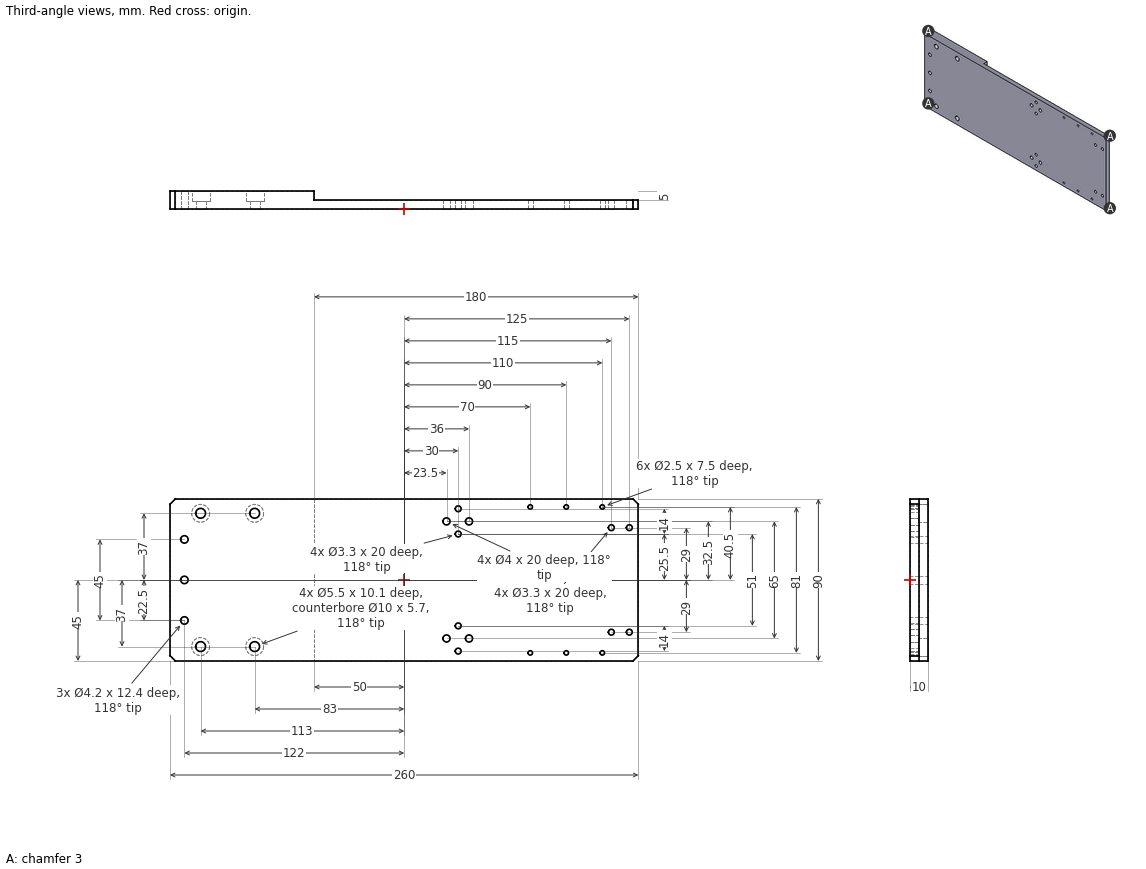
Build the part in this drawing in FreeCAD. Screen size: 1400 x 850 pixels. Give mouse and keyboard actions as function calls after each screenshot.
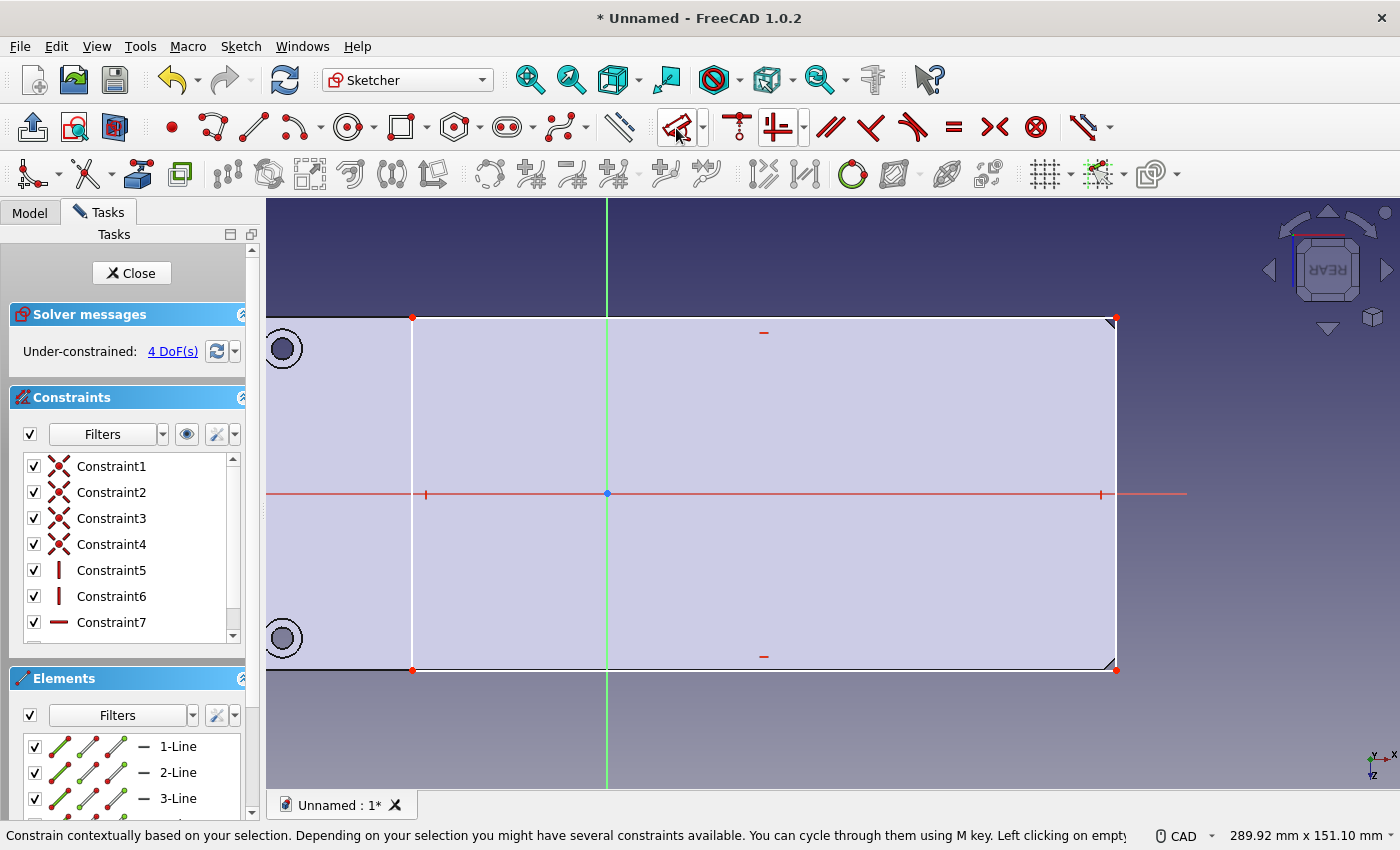
click(412, 424)
click(378, 413)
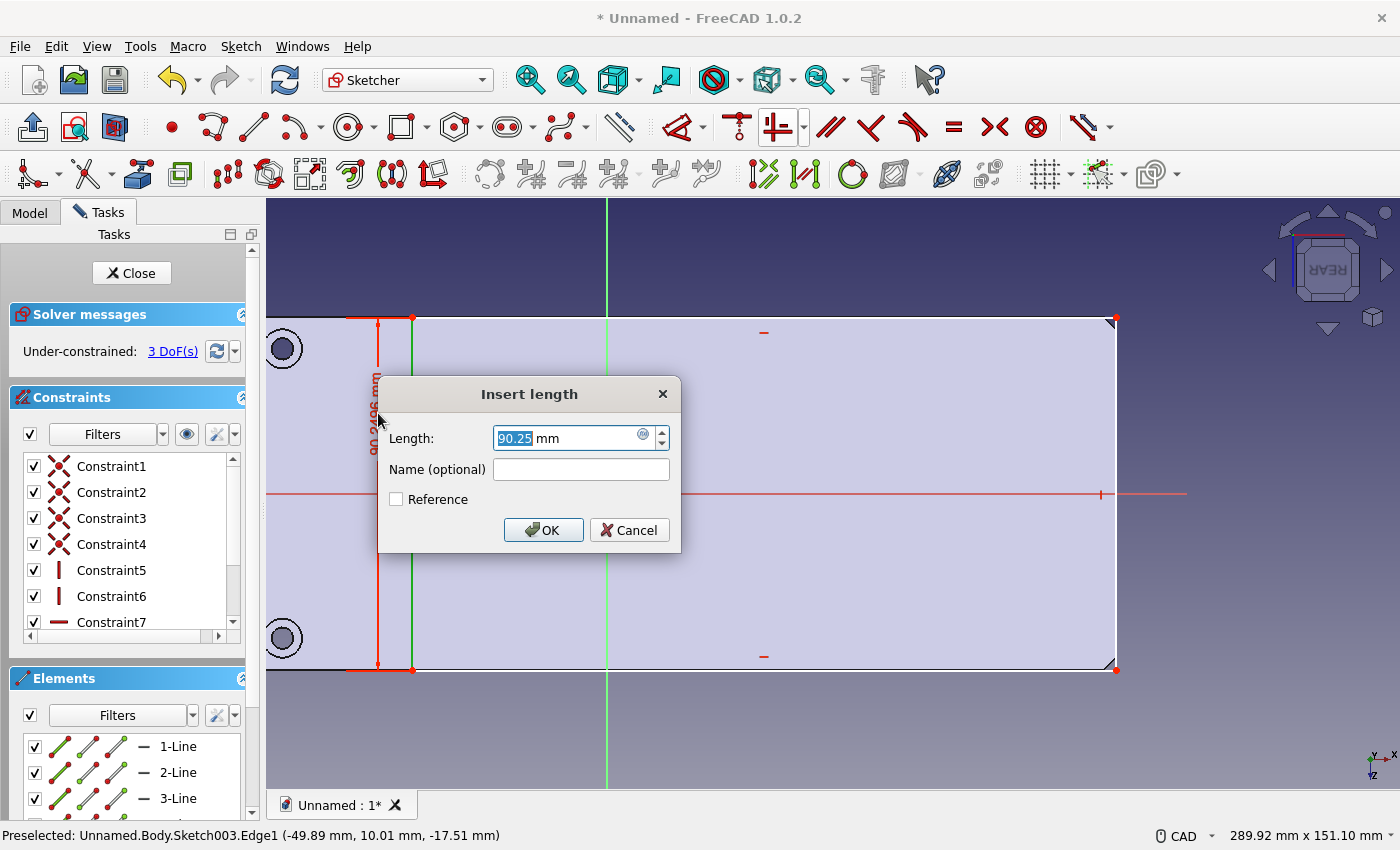
text(90)
key(Return)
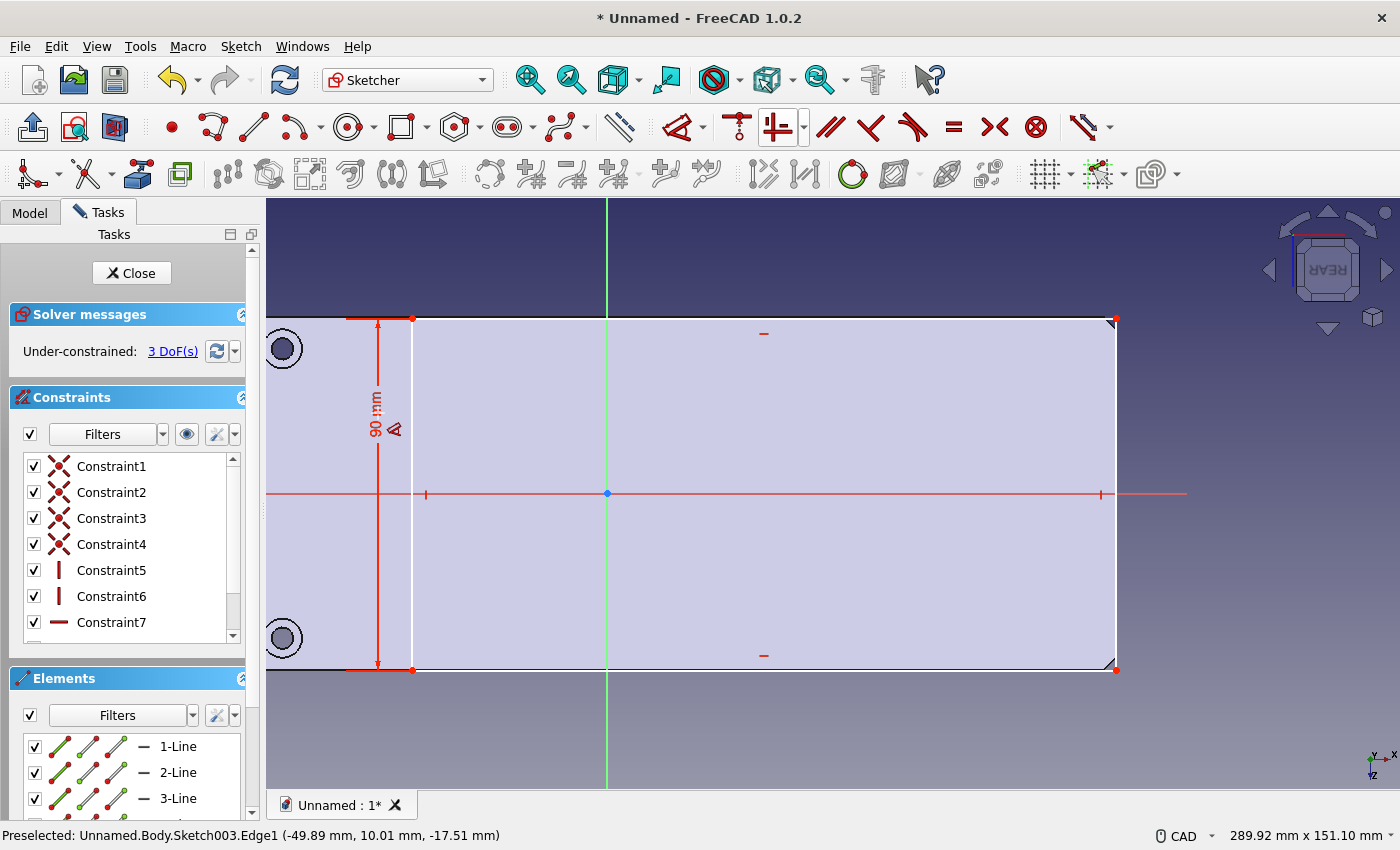
click(623, 671)
click(764, 705)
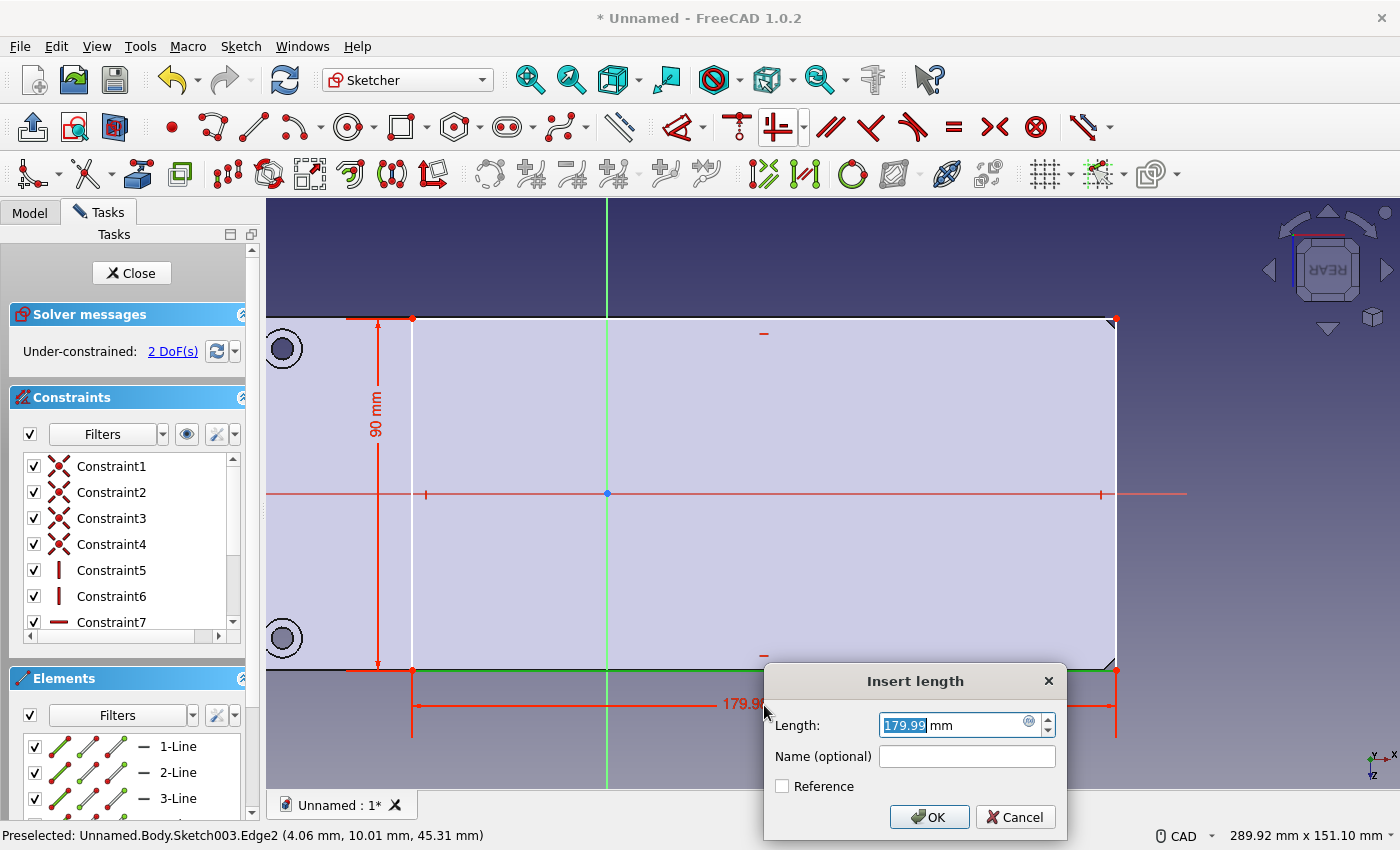
text(180)
key(Return)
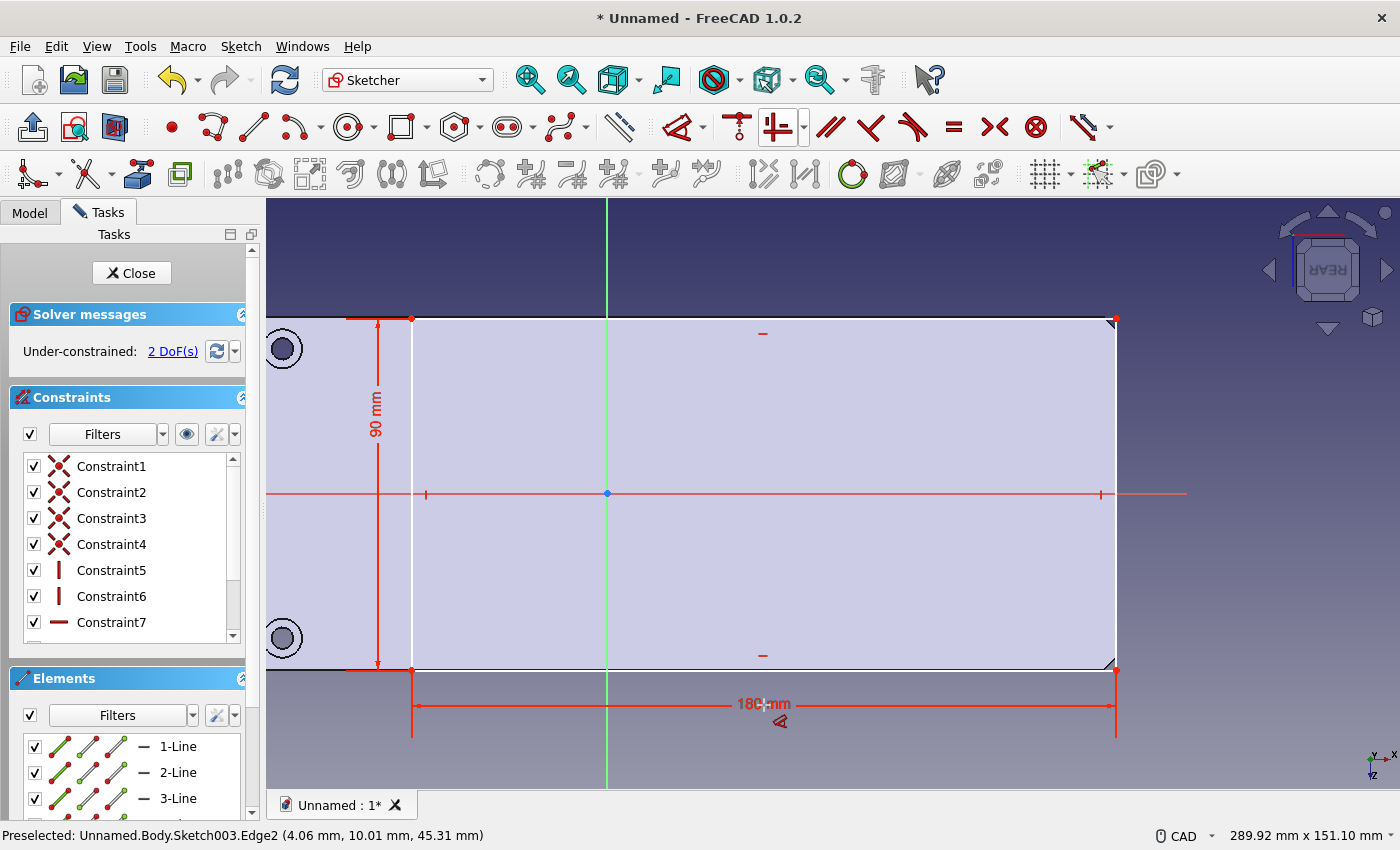
click(412, 319)
click(510, 285)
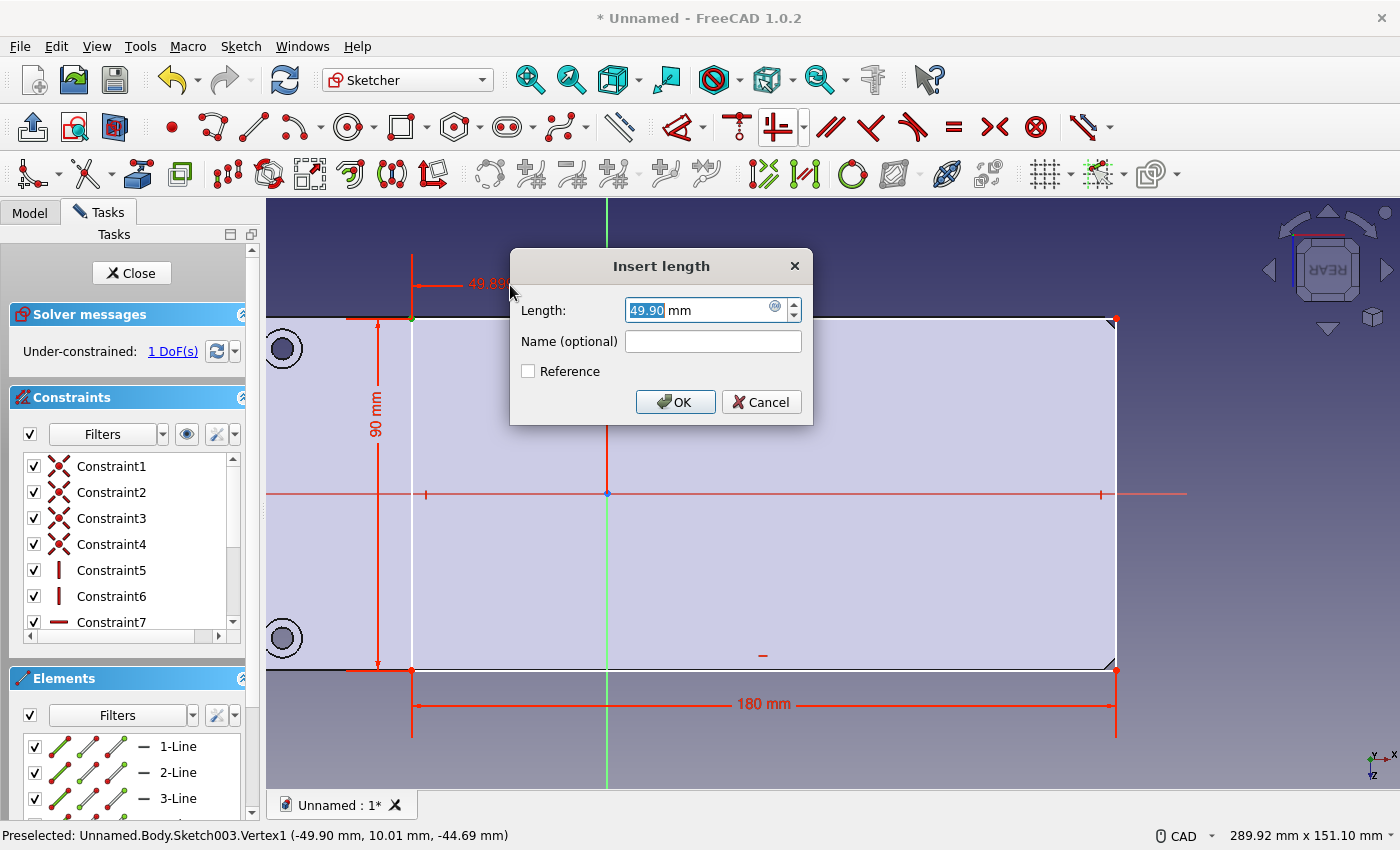
text(50)
key(Return)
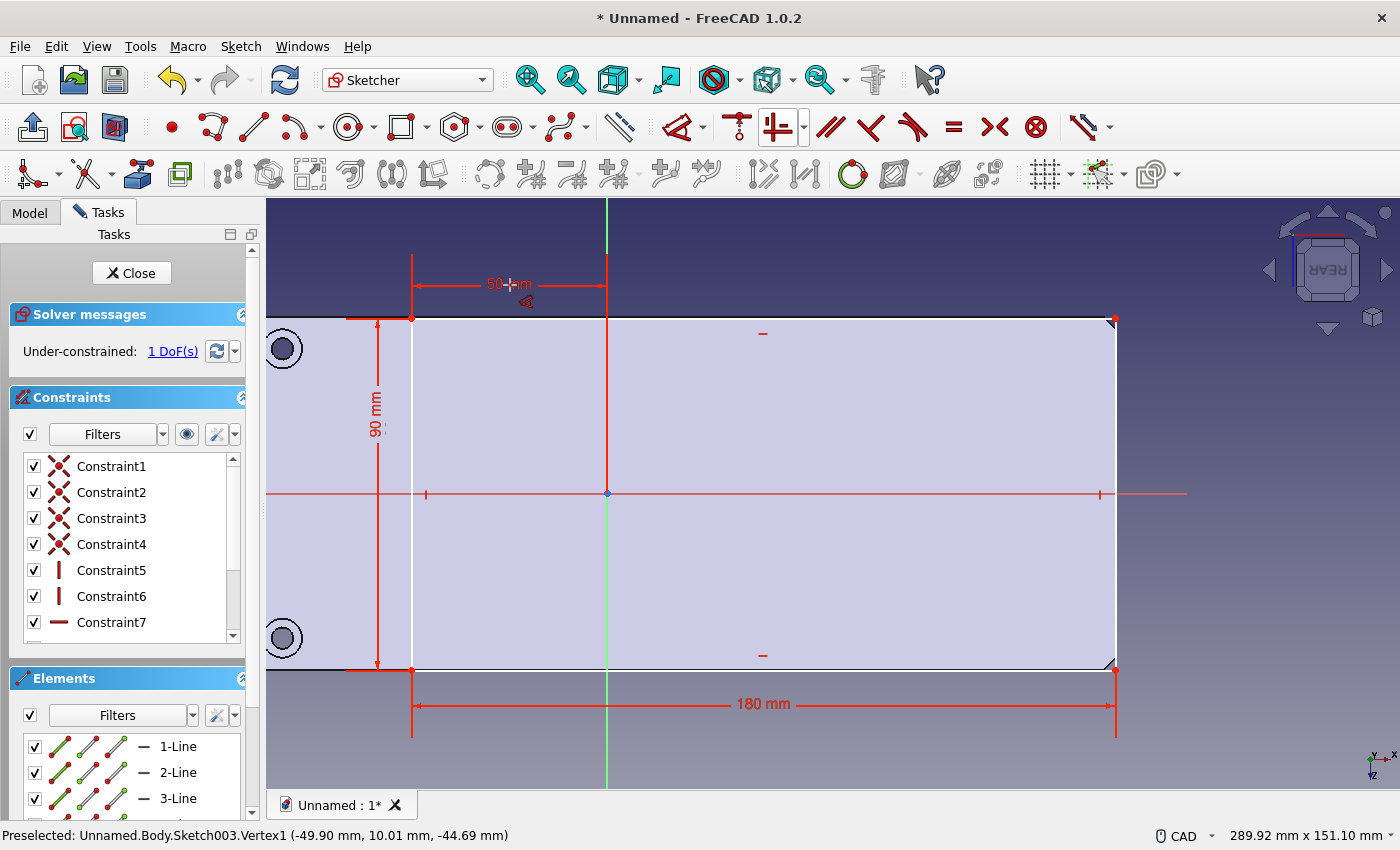
click(412, 319)
click(378, 366)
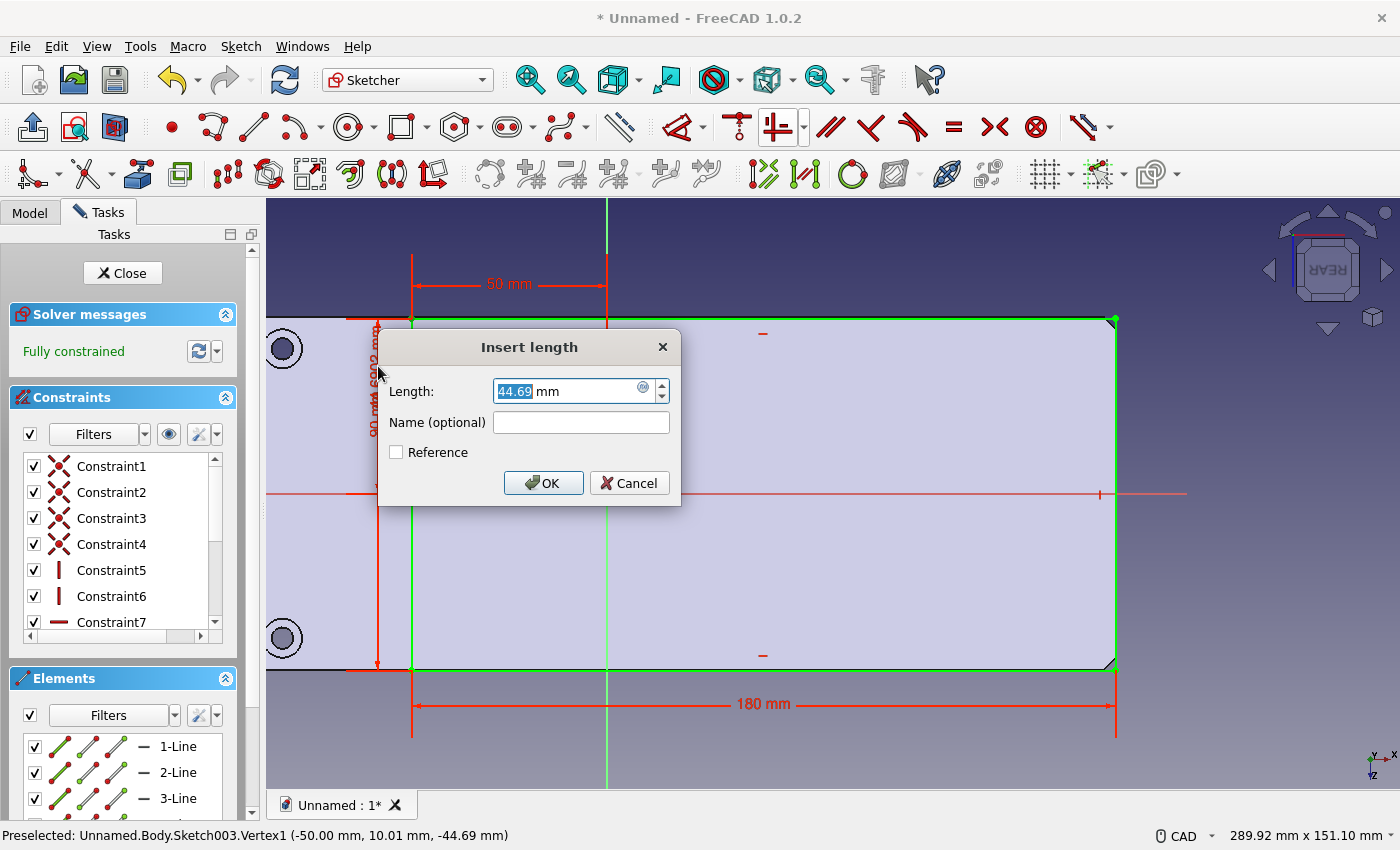
text(45)
key(Return)
key(Escape)